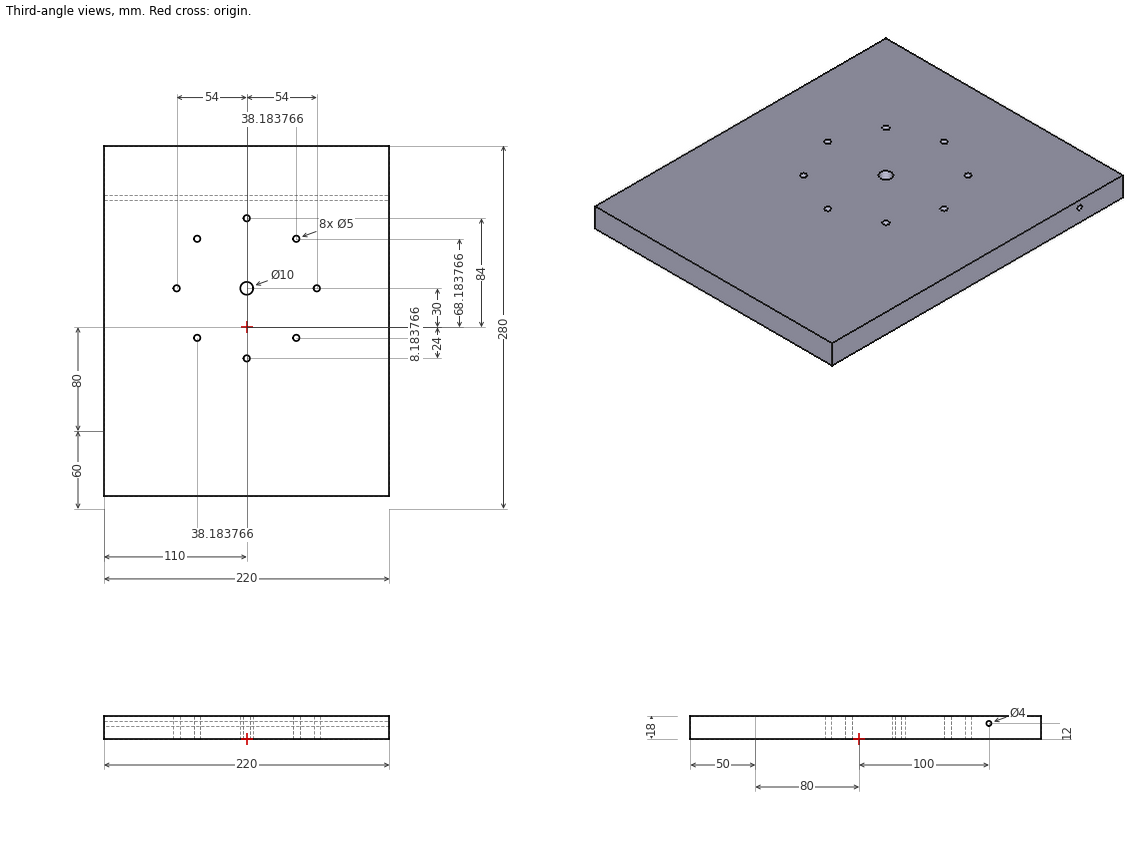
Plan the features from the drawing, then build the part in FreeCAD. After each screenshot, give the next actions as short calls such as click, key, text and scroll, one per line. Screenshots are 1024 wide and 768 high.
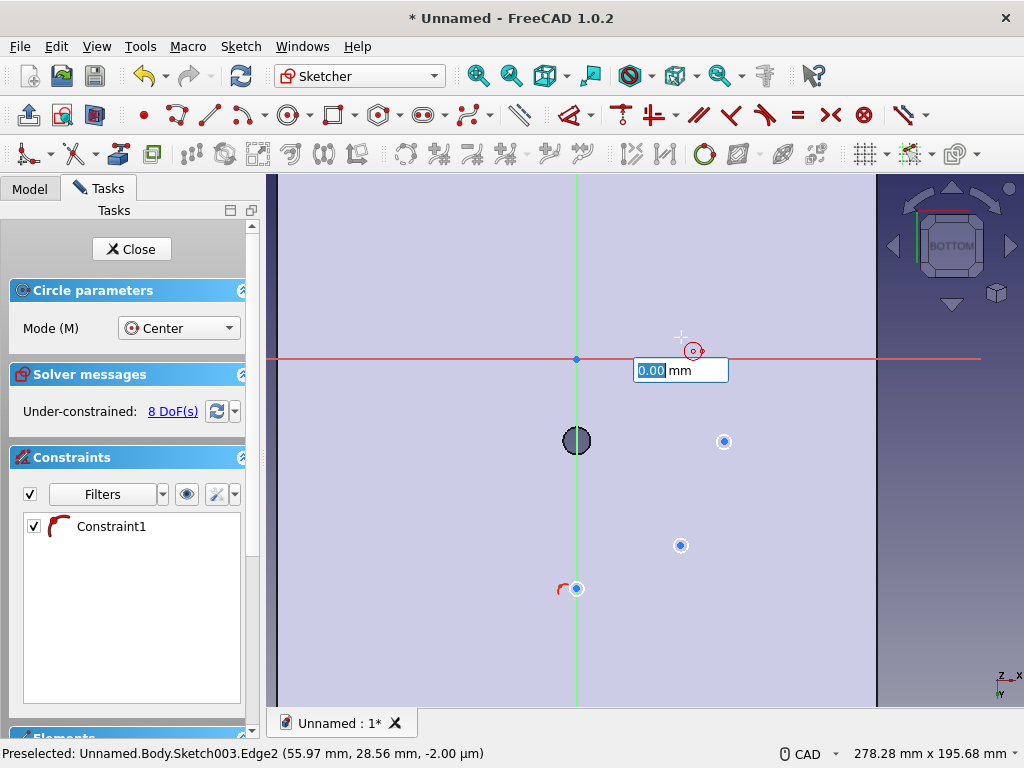
scroll(686, 332, up, 5)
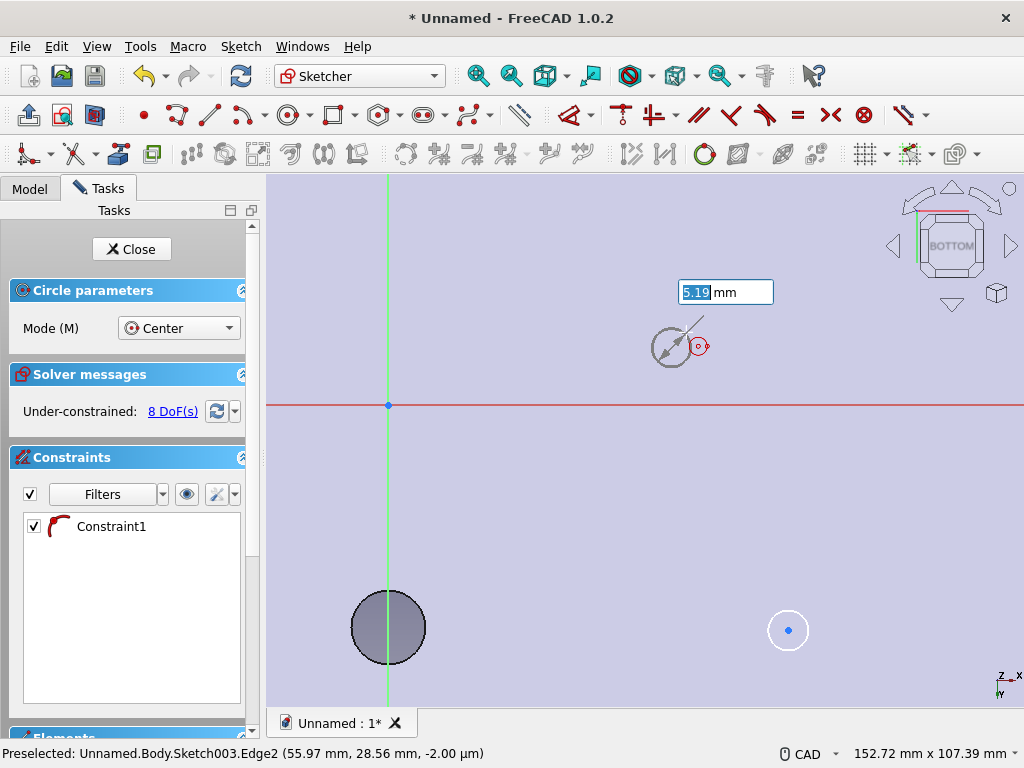
click(684, 332)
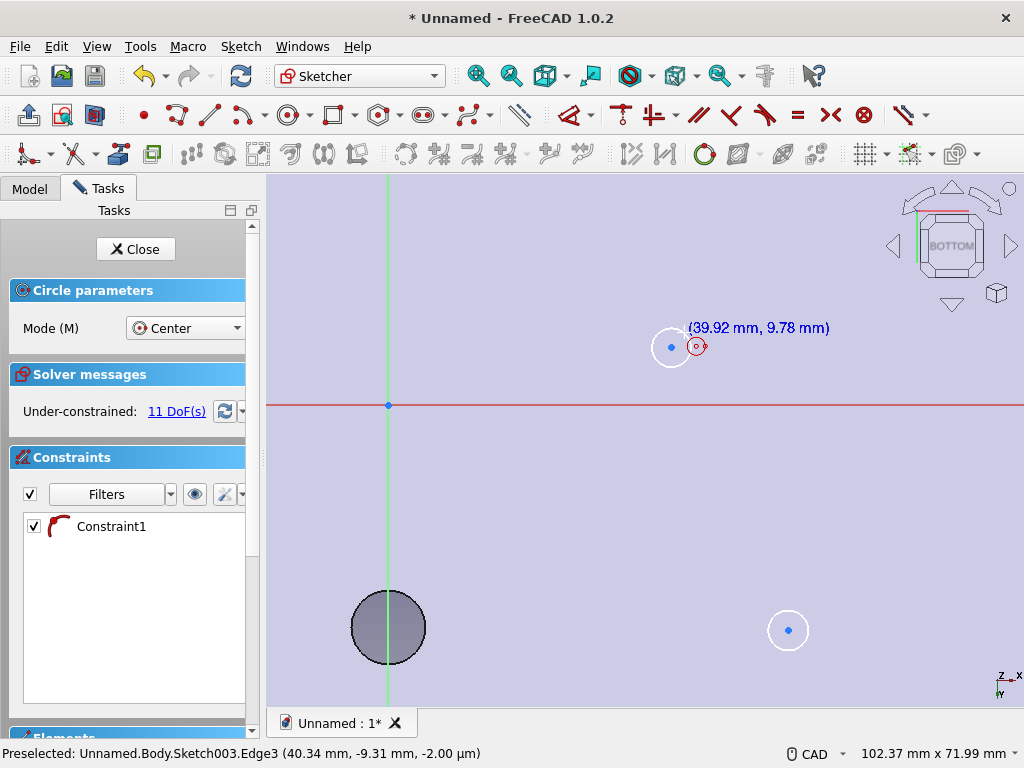
scroll(388, 228, up, 2)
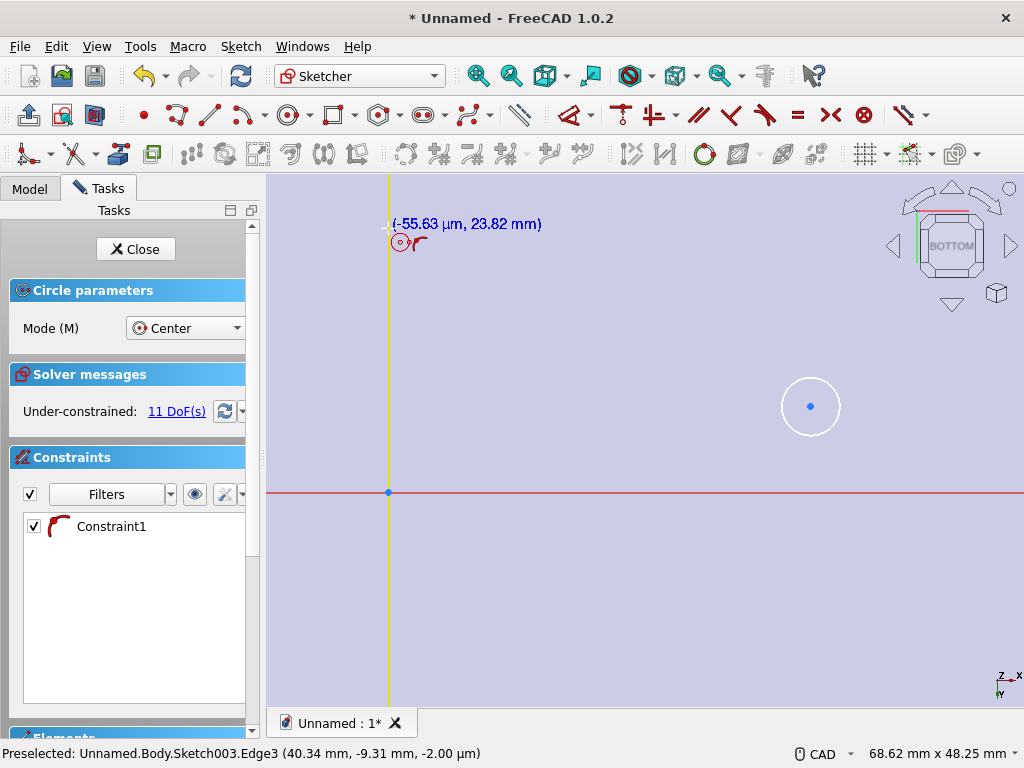
scroll(638, 315, down, 7)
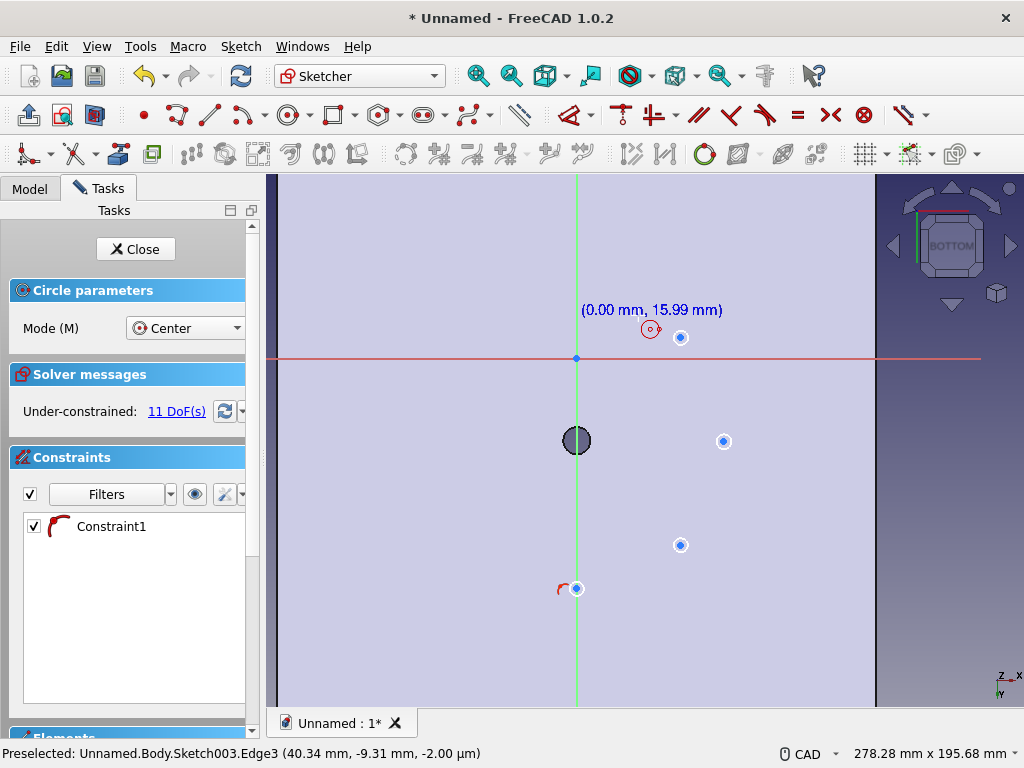
click(577, 294)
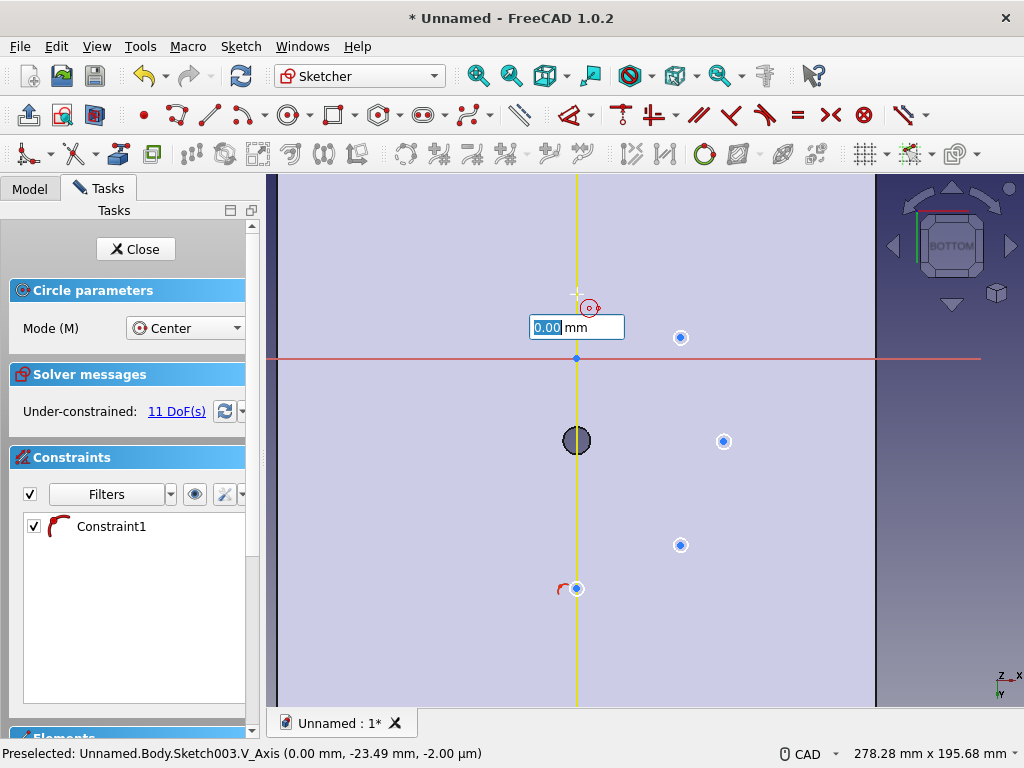
scroll(583, 291, up, 5)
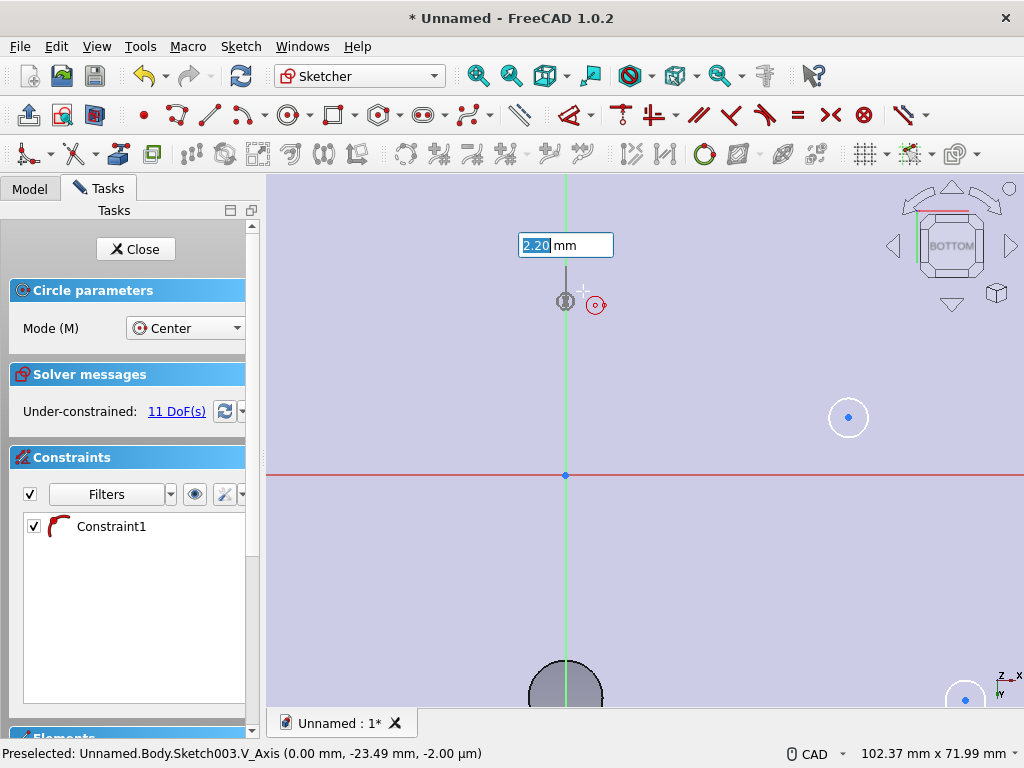
click(583, 291)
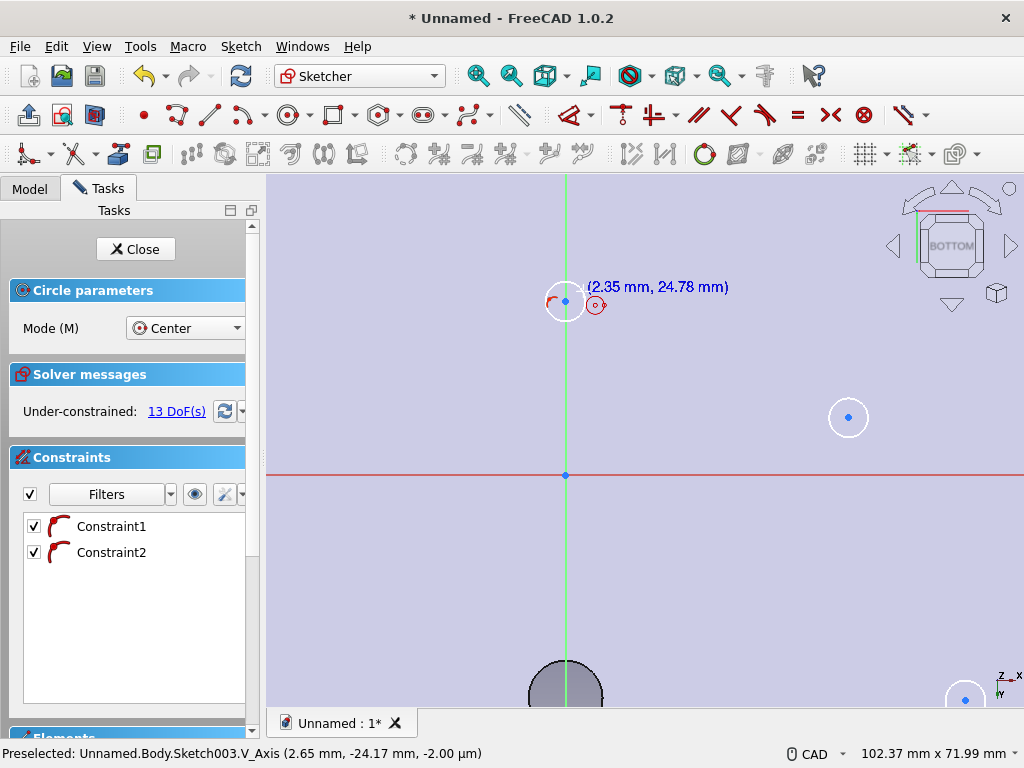
scroll(583, 291, down, 5)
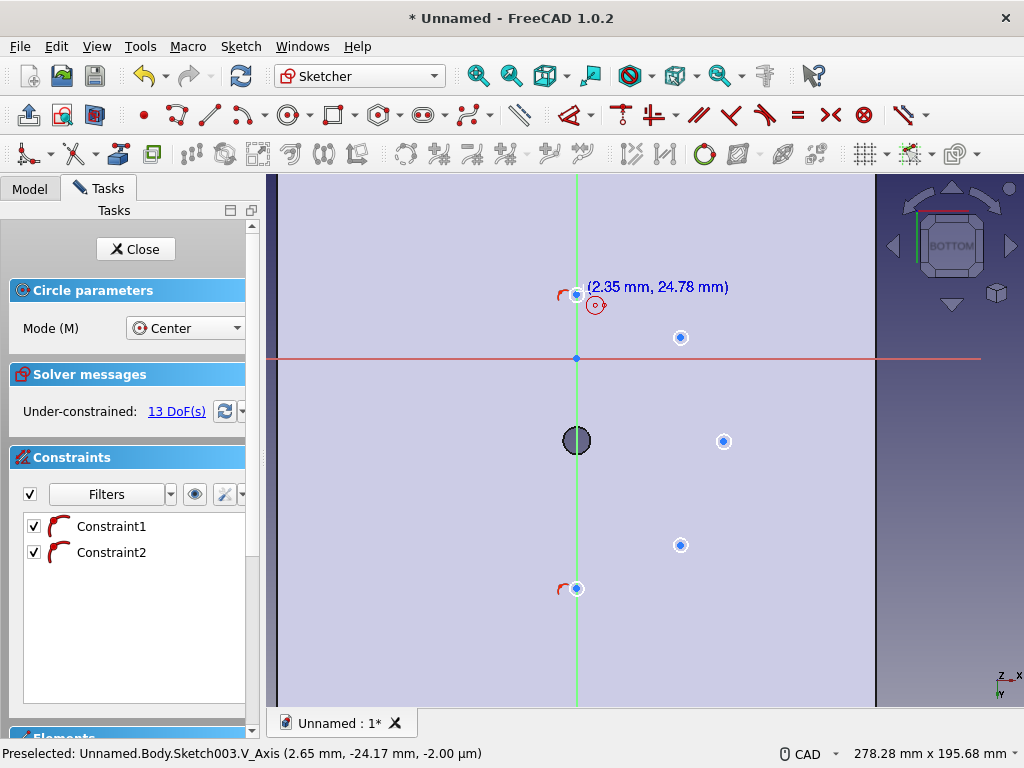
scroll(473, 337, up, 7)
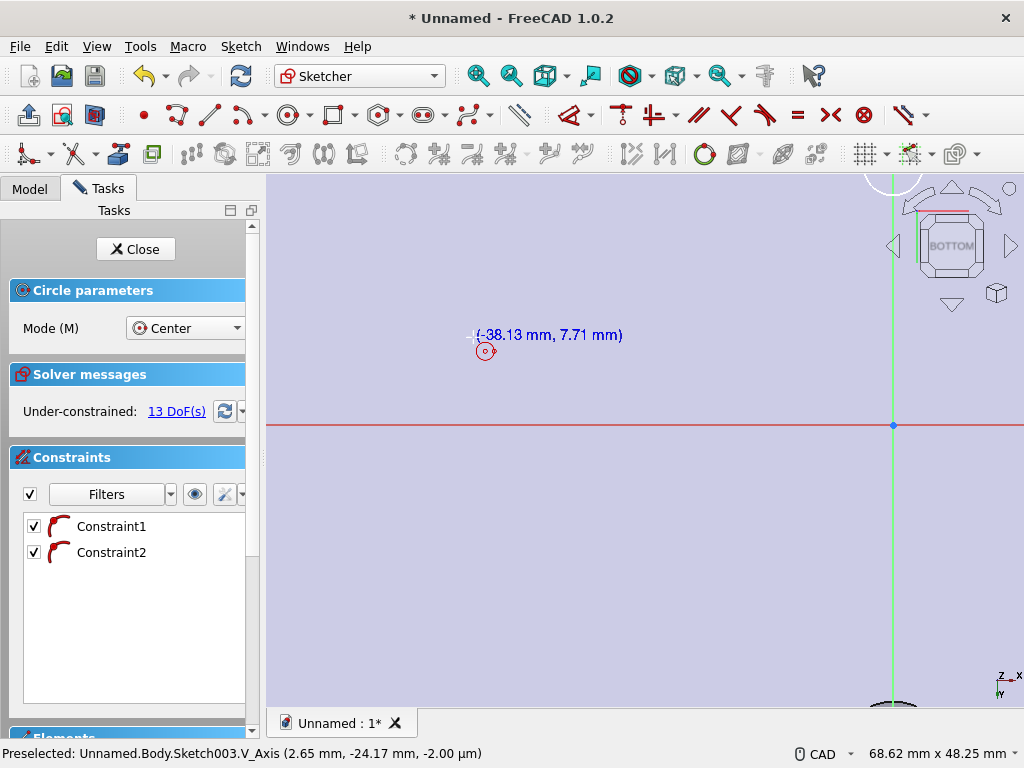
scroll(473, 337, down, 7)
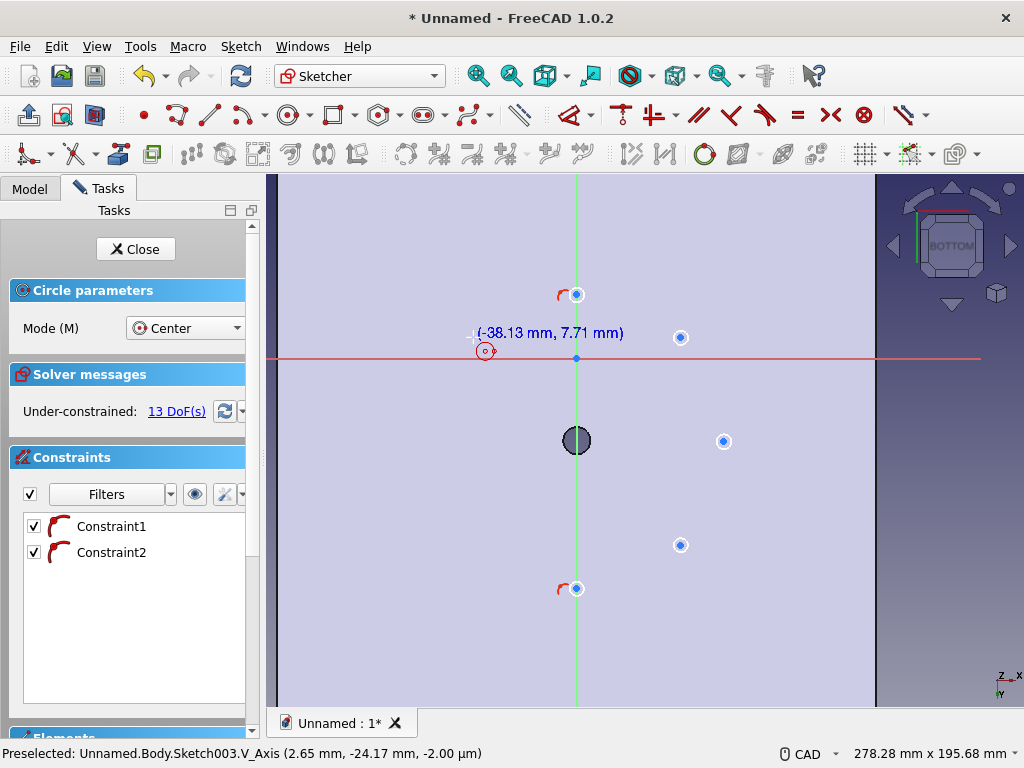
click(473, 337)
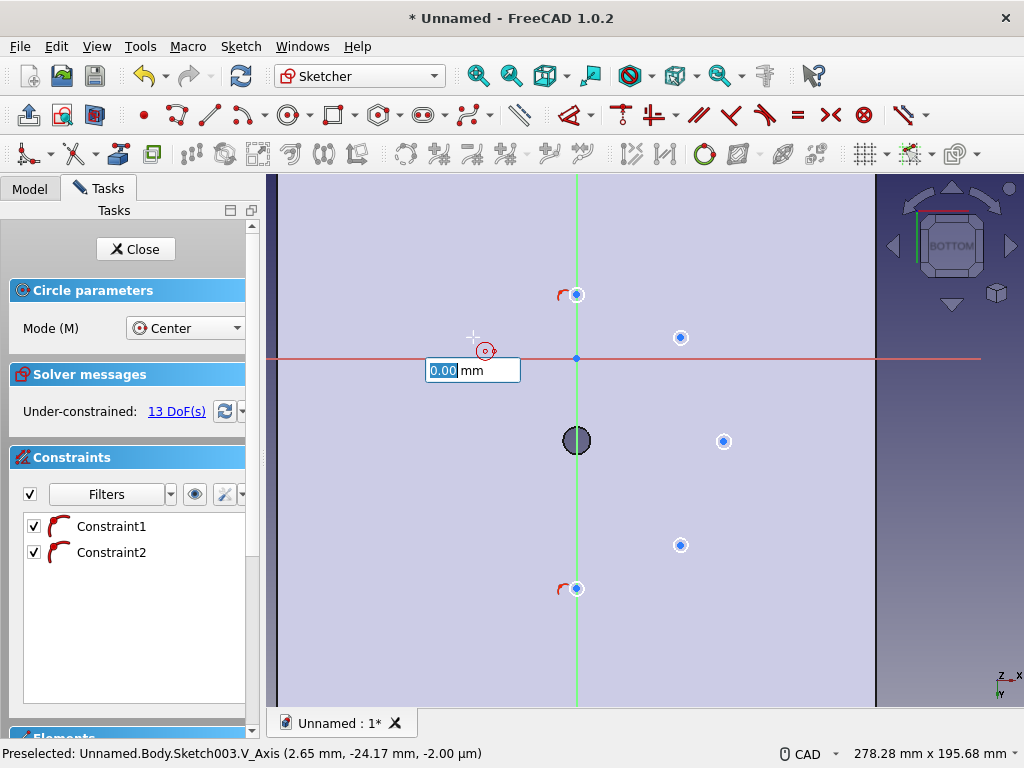
scroll(478, 332, up, 5)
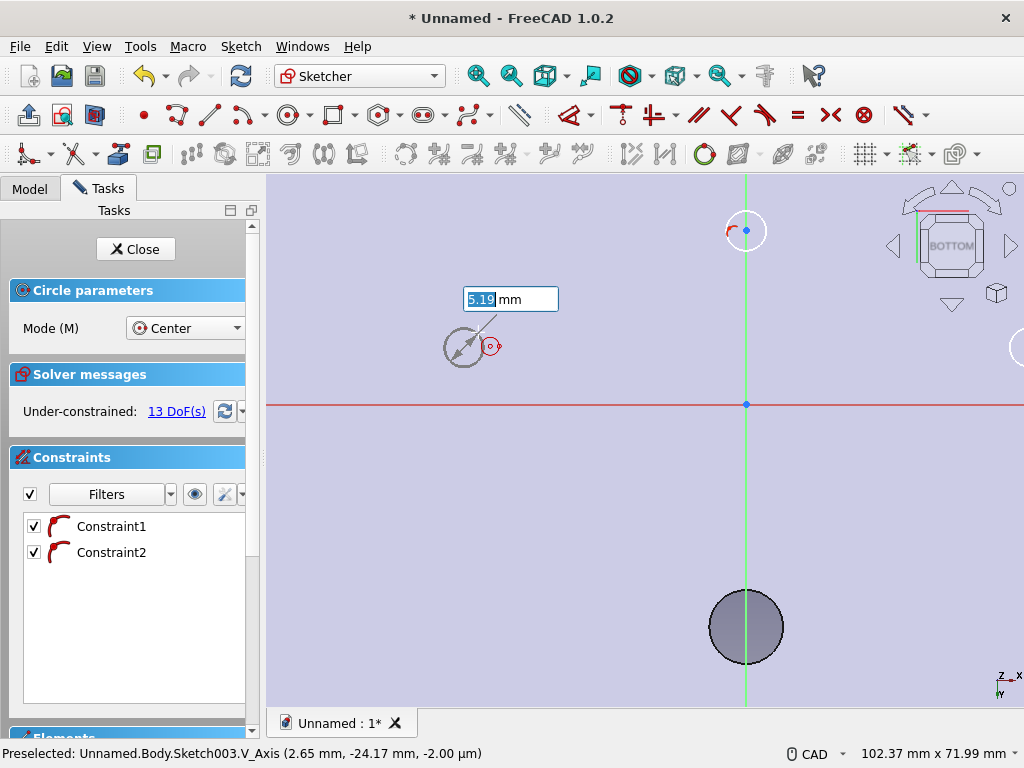
click(477, 331)